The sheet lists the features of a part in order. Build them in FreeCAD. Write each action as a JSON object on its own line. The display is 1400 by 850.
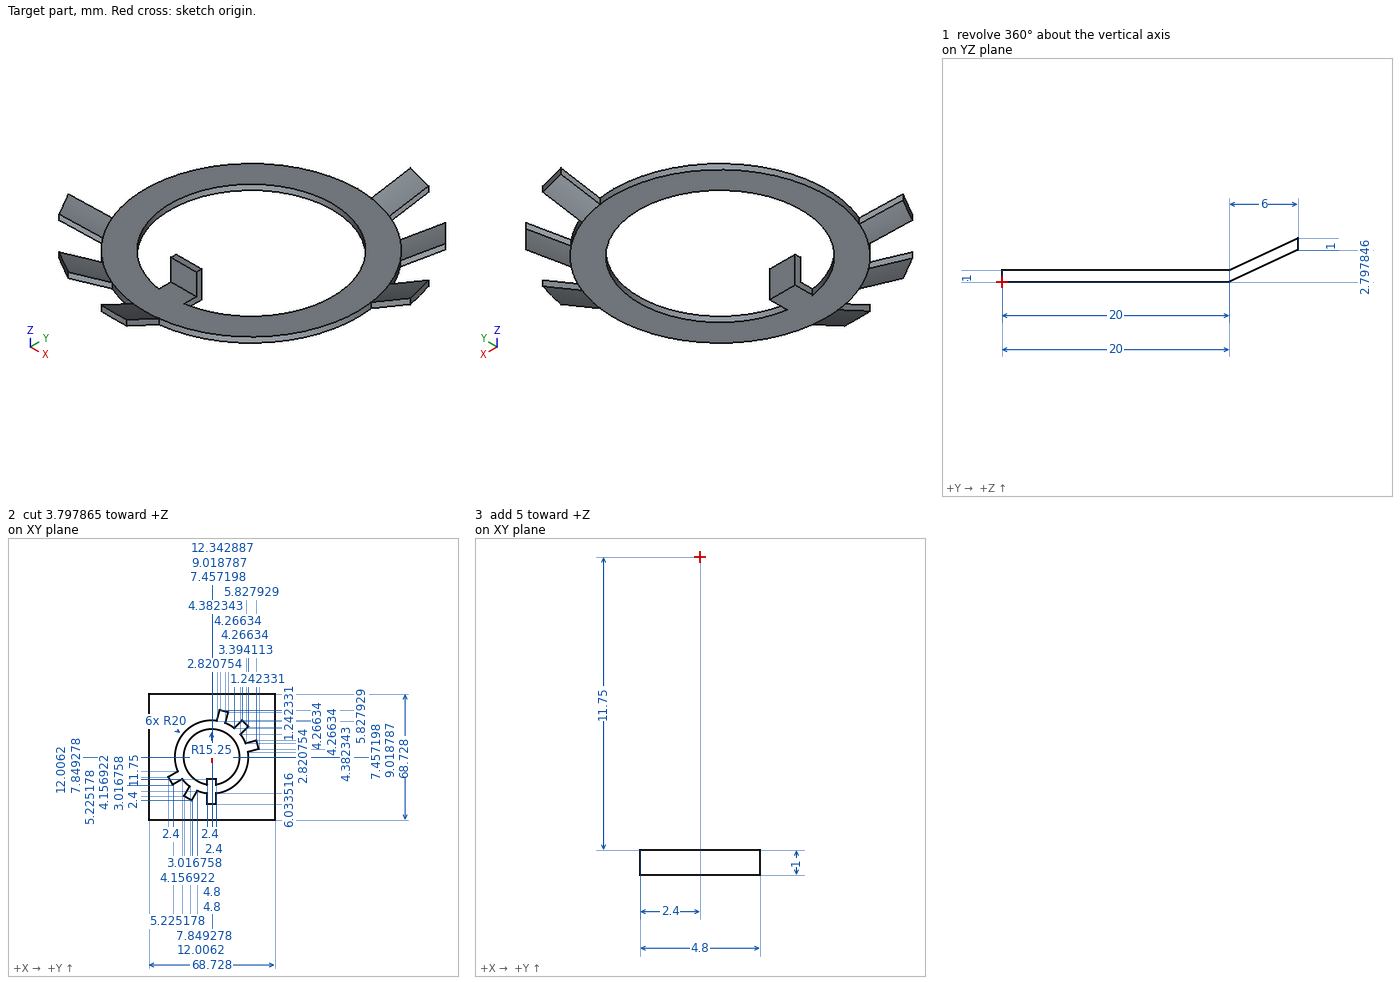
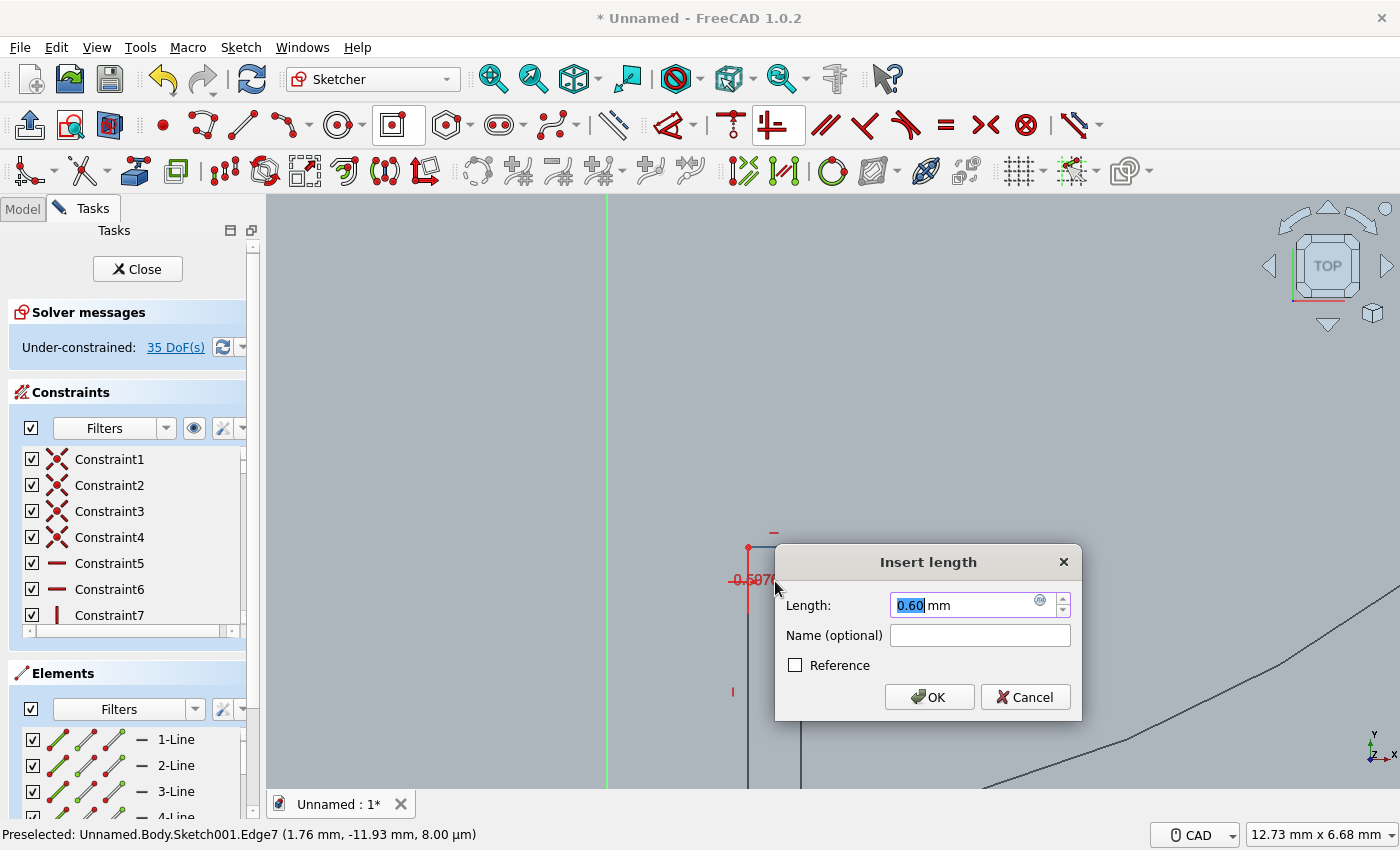
{"action": "type", "text": "4.8"}
{"action": "key", "text": "Return"}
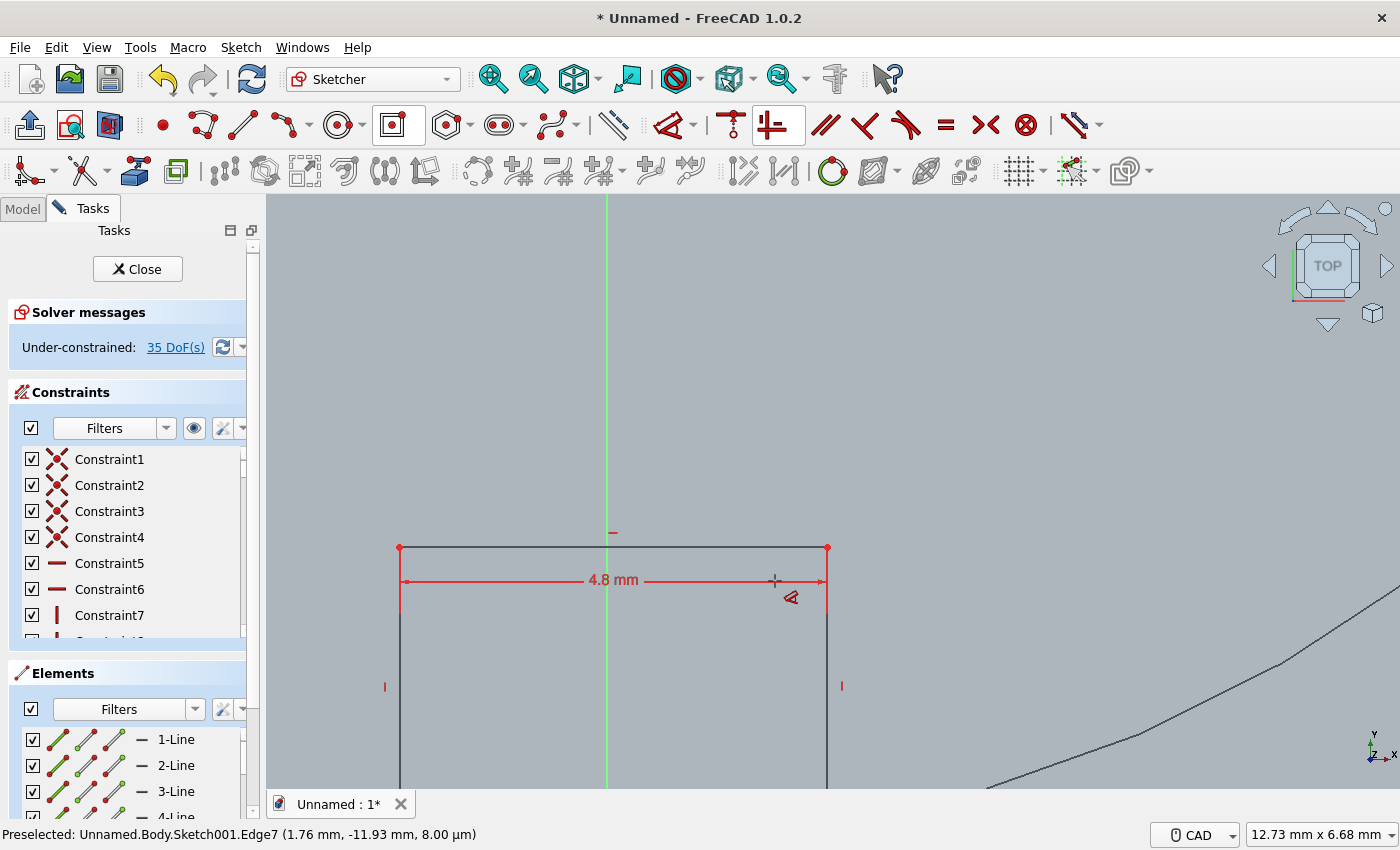
{"action": "scroll", "coordinate": [775, 557], "scroll_direction": "down", "scroll_amount": 14}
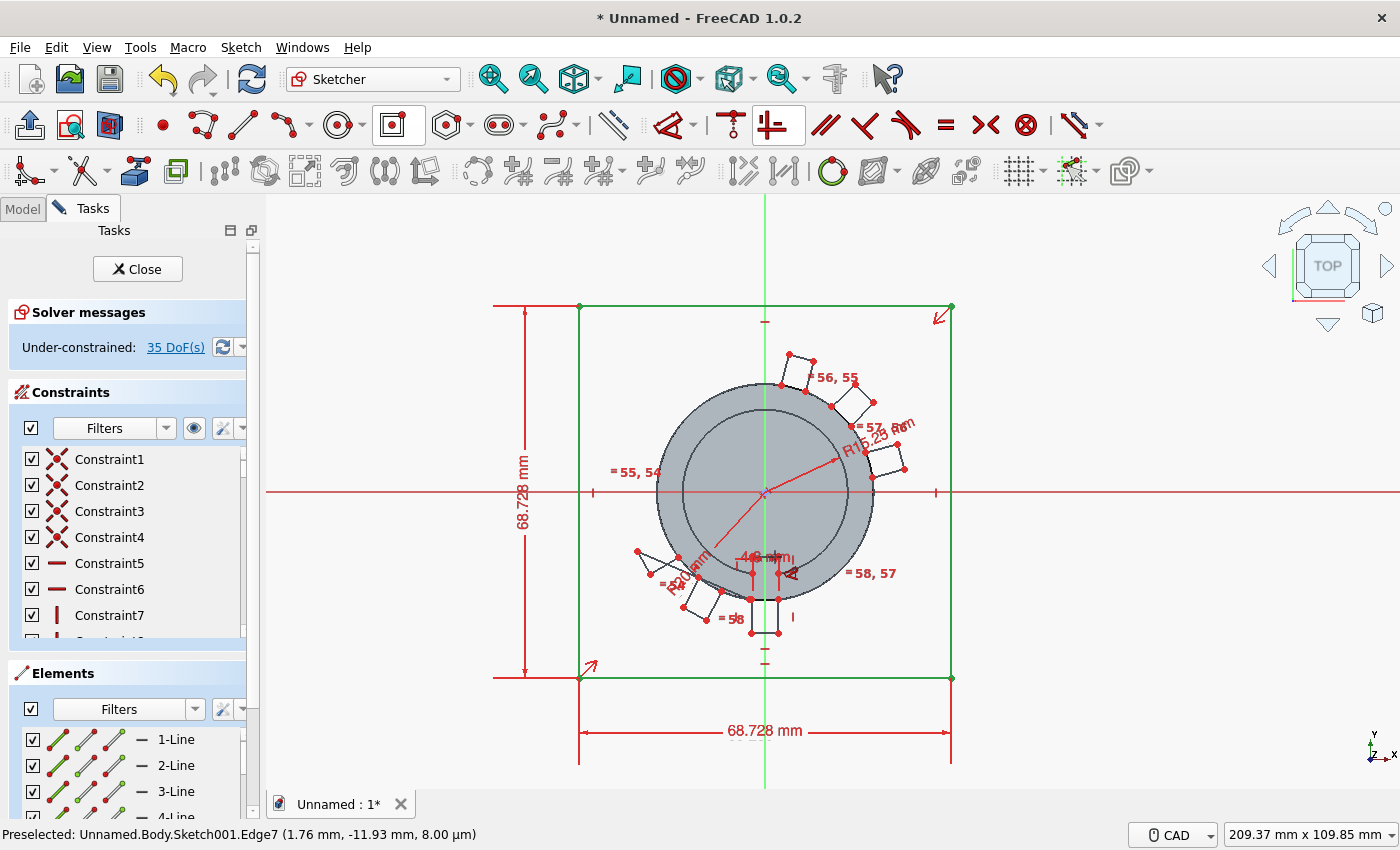
{"action": "scroll", "coordinate": [770, 633], "scroll_direction": "up", "scroll_amount": 5}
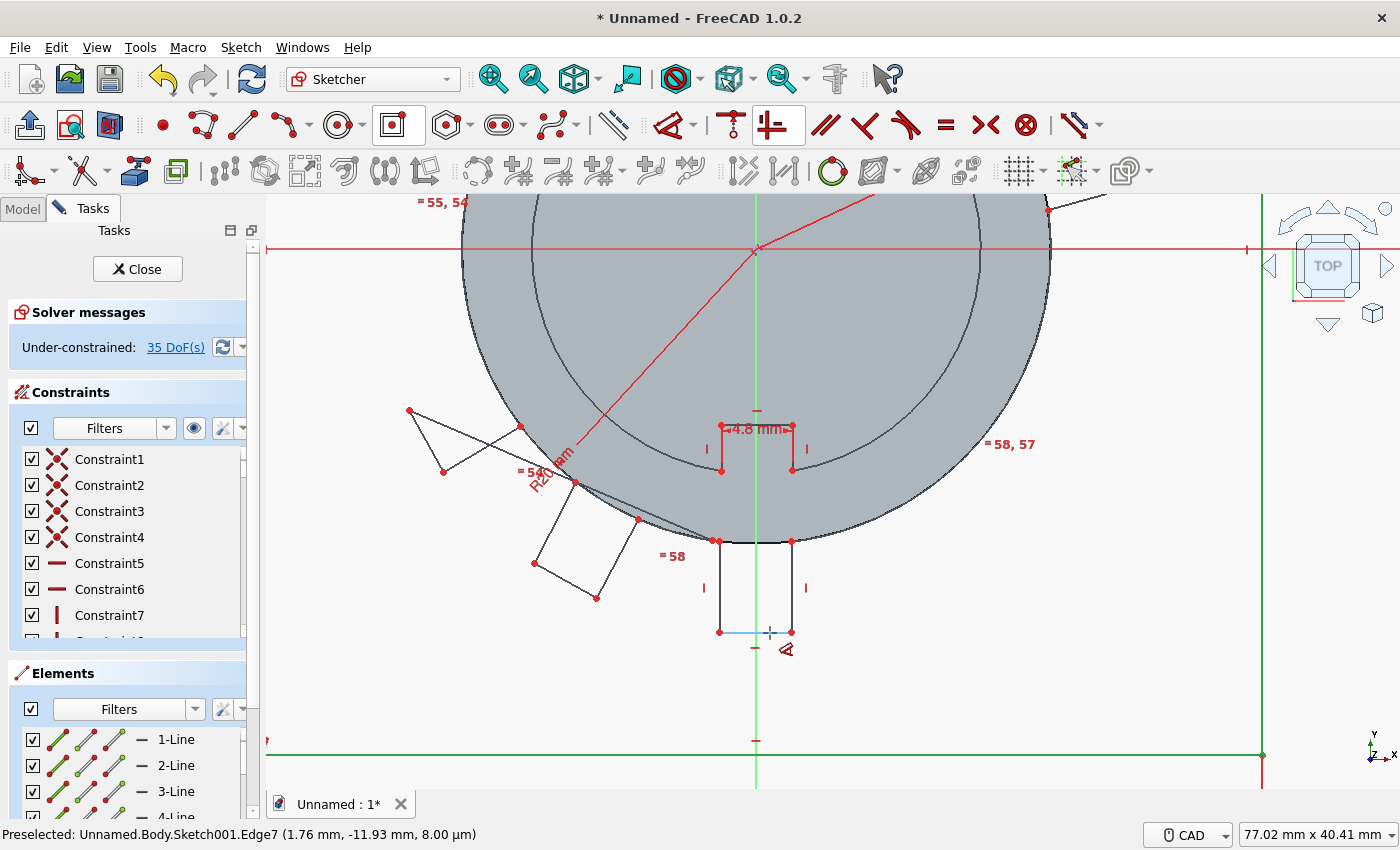
{"action": "left_click", "coordinate": [770, 633]}
{"action": "left_click", "coordinate": [739, 667]}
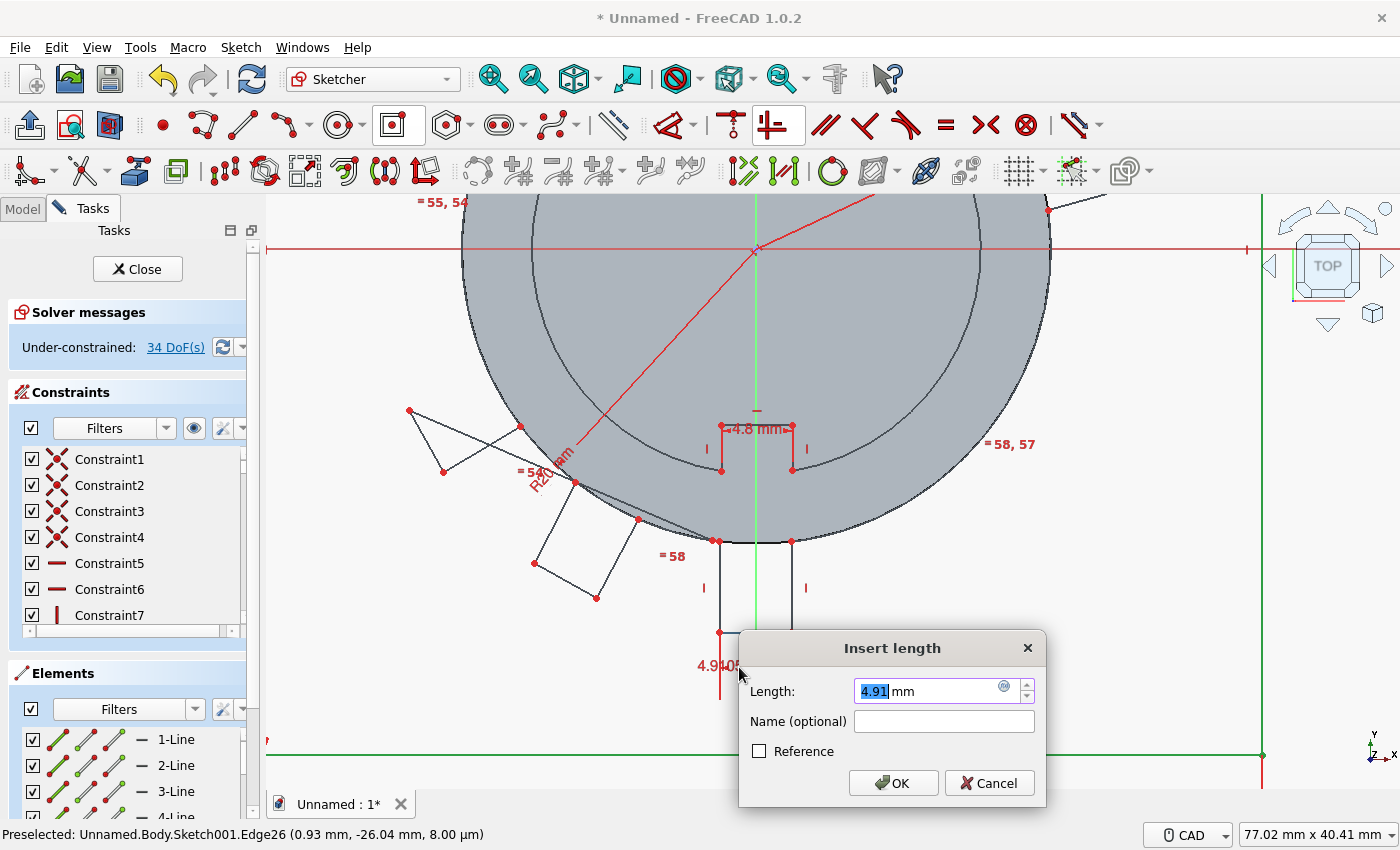
{"action": "type", "text": "4.8"}
{"action": "key", "text": "Return"}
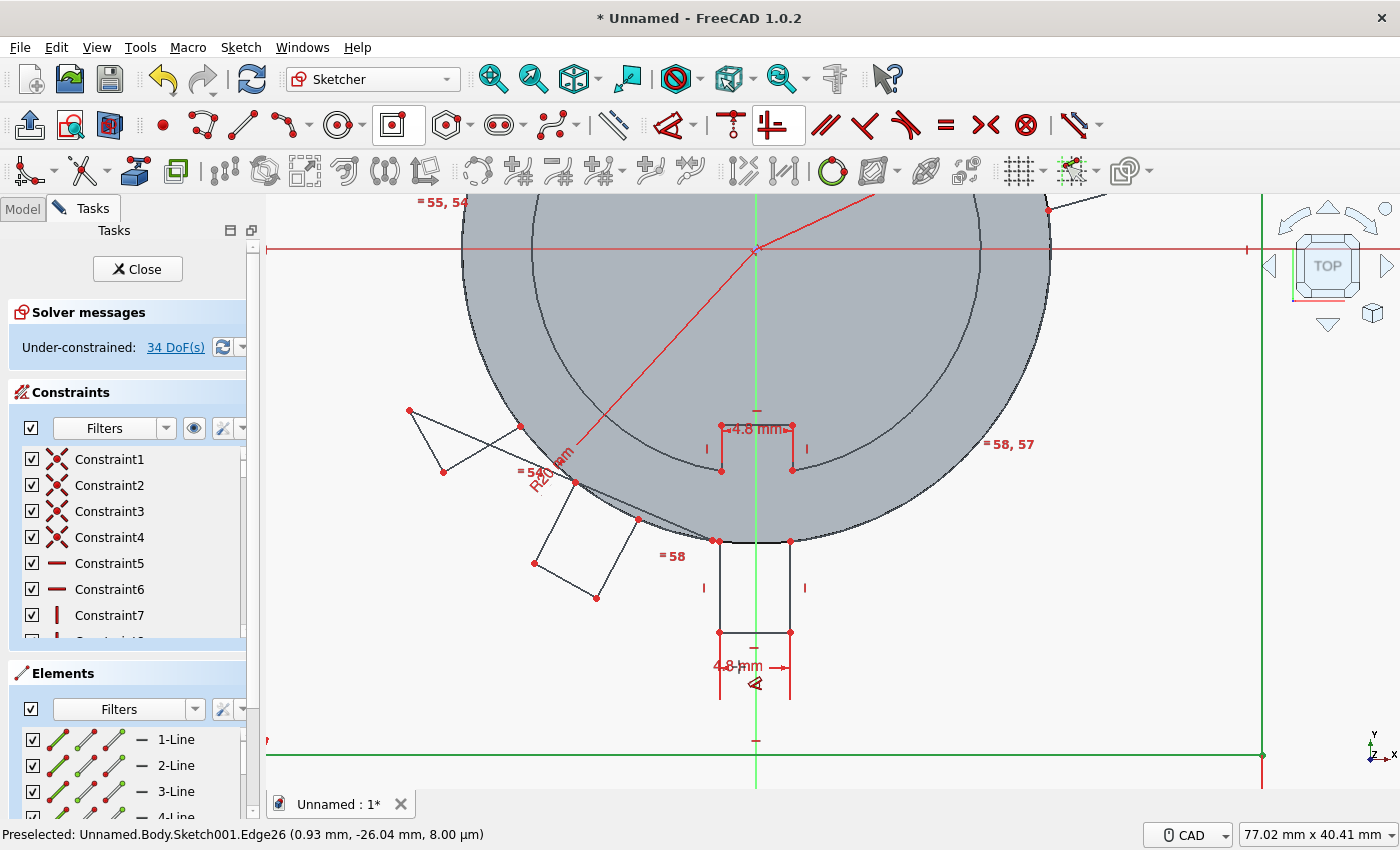
{"action": "left_click", "coordinate": [722, 471]}
{"action": "left_click", "coordinate": [739, 505]}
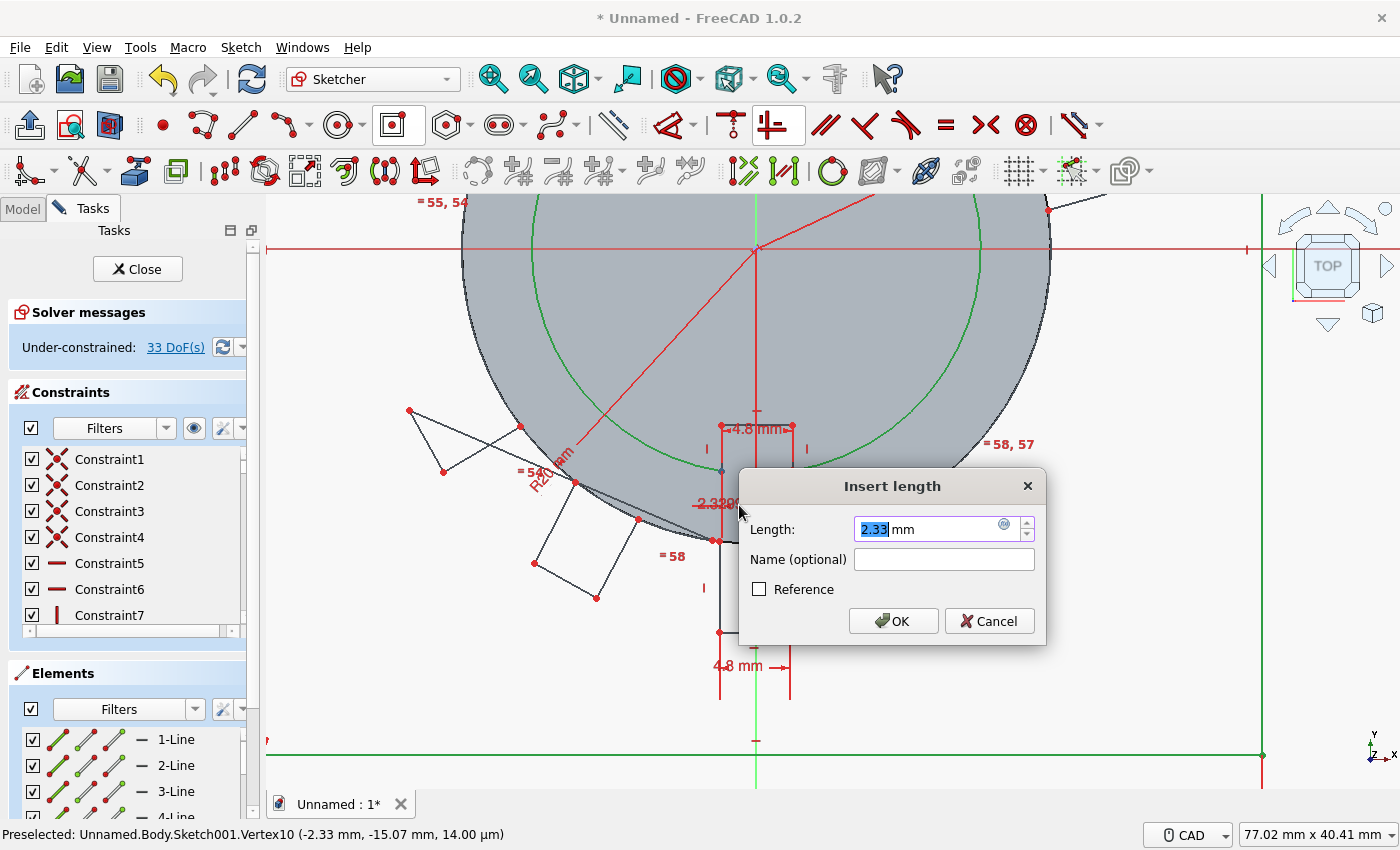
{"action": "type", "text": "2.4"}
{"action": "key", "text": "Return"}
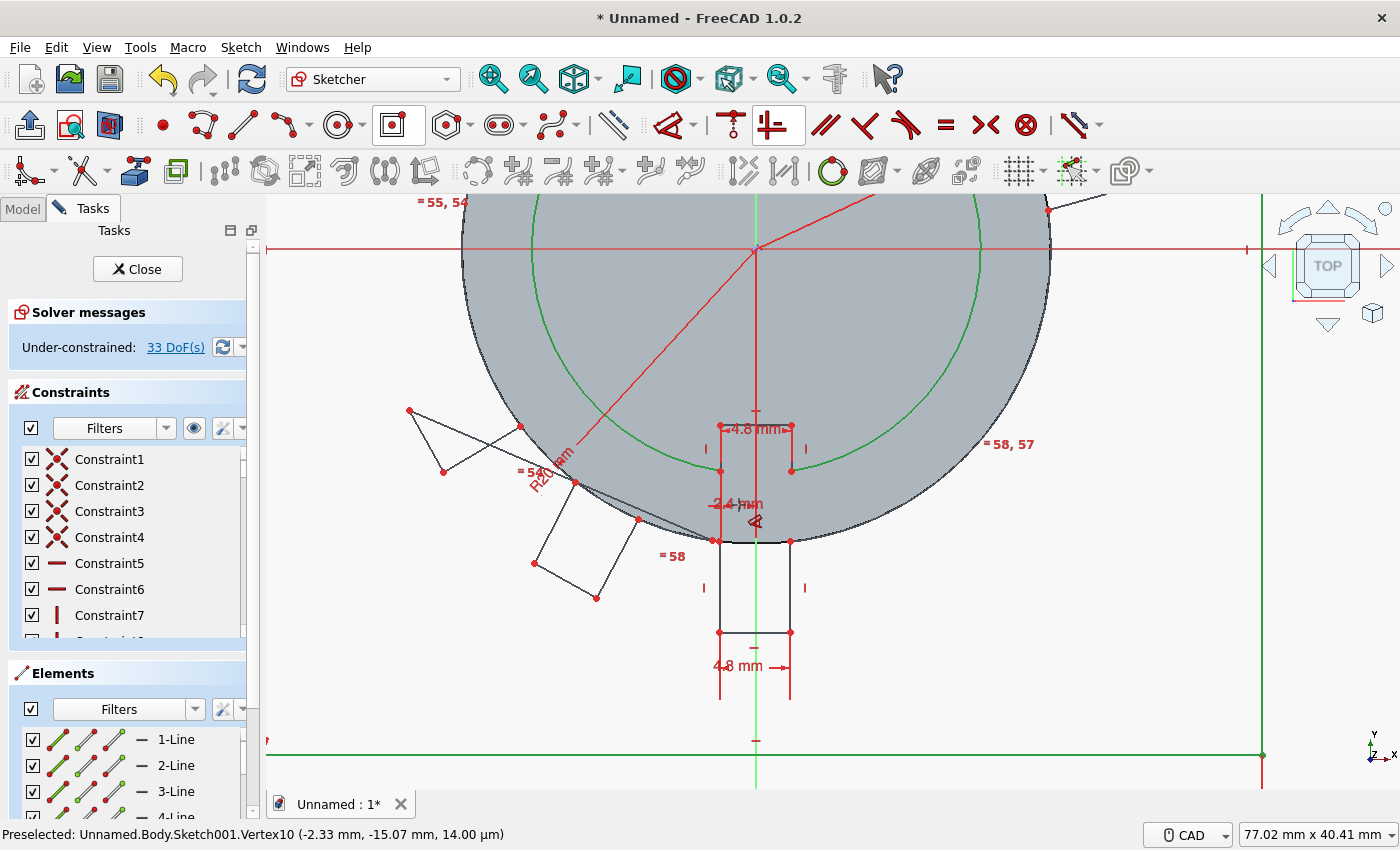
{"action": "left_click", "coordinate": [790, 542]}
{"action": "left_click", "coordinate": [773, 576]}